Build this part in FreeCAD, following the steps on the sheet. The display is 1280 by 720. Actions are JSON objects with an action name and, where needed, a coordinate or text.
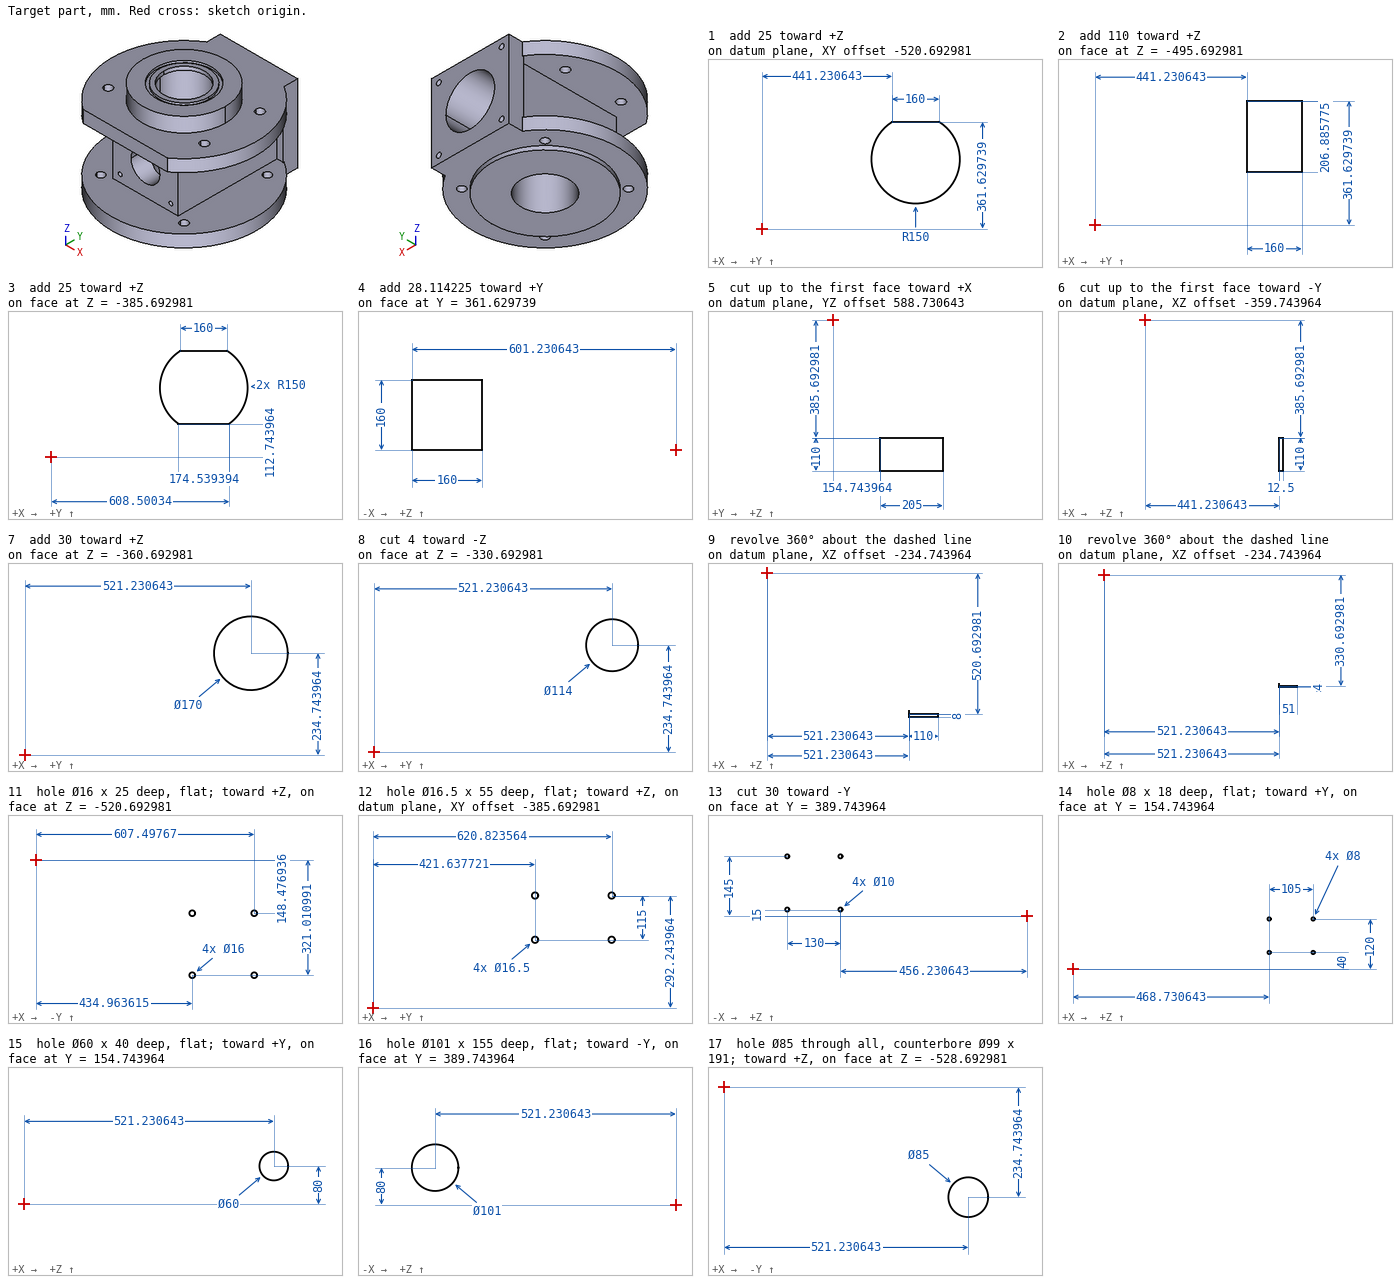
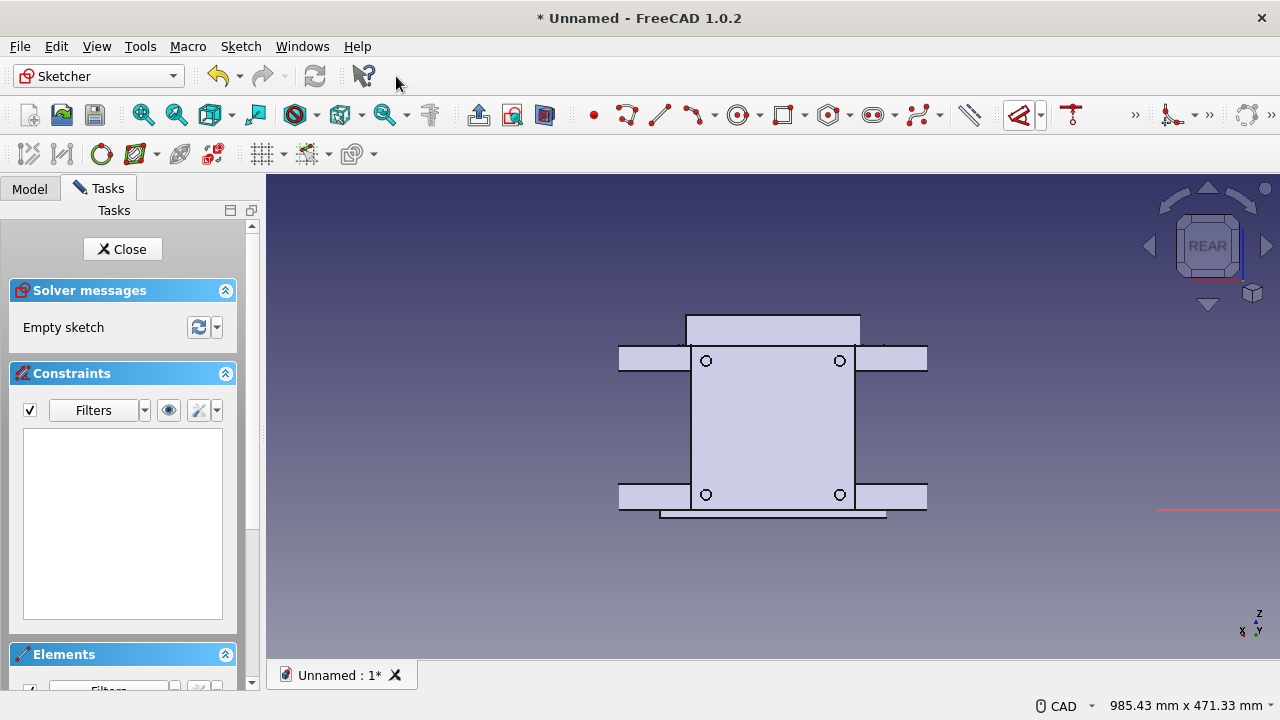
{"action": "scroll", "coordinate": [813, 434], "scroll_direction": "up", "scroll_amount": 5}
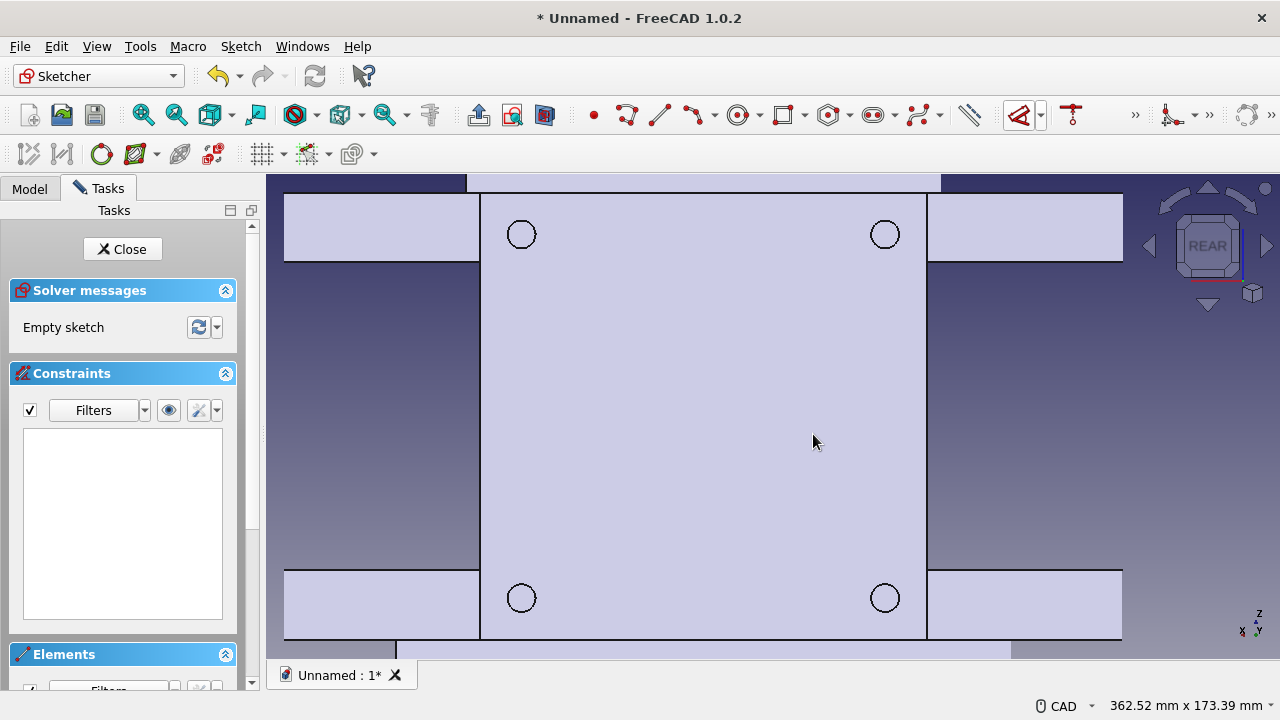
{"action": "left_click", "coordinate": [738, 116]}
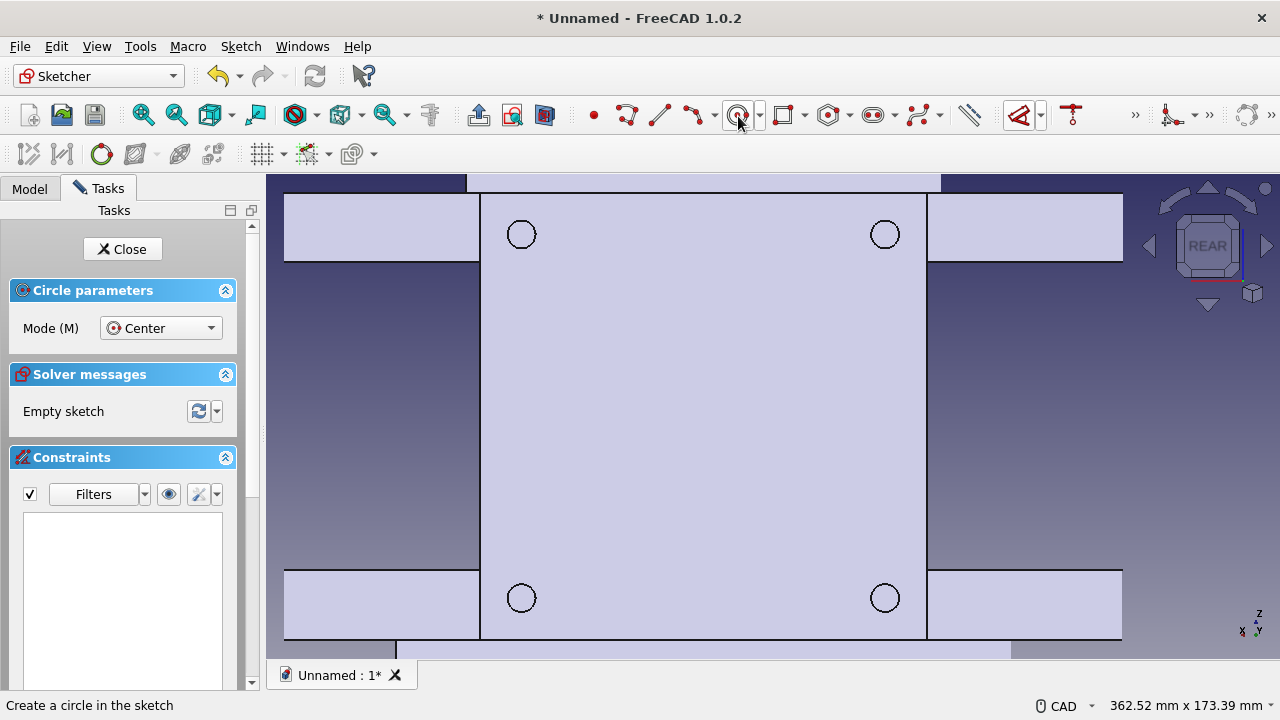
{"action": "left_click", "coordinate": [703, 416]}
{"action": "left_click", "coordinate": [803, 316]}
{"action": "key", "text": "Escape"}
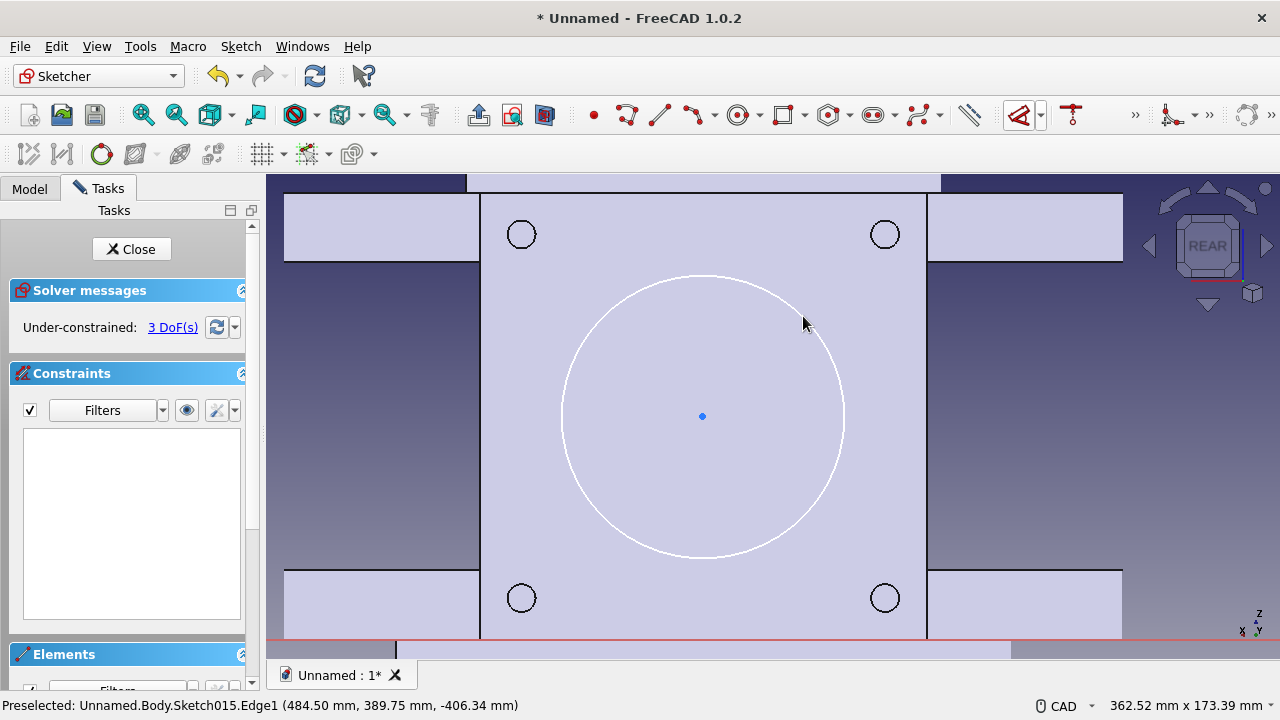
{"action": "left_click", "coordinate": [803, 317]}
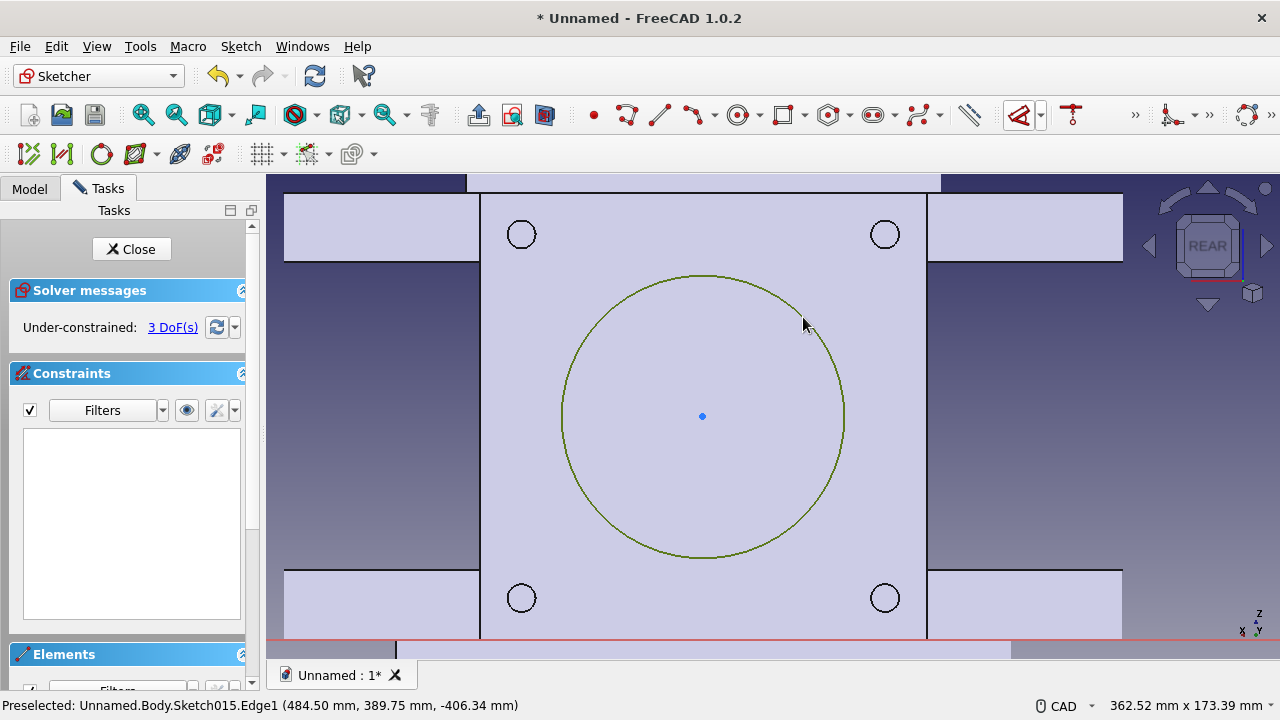
{"action": "left_click", "coordinate": [1040, 116]}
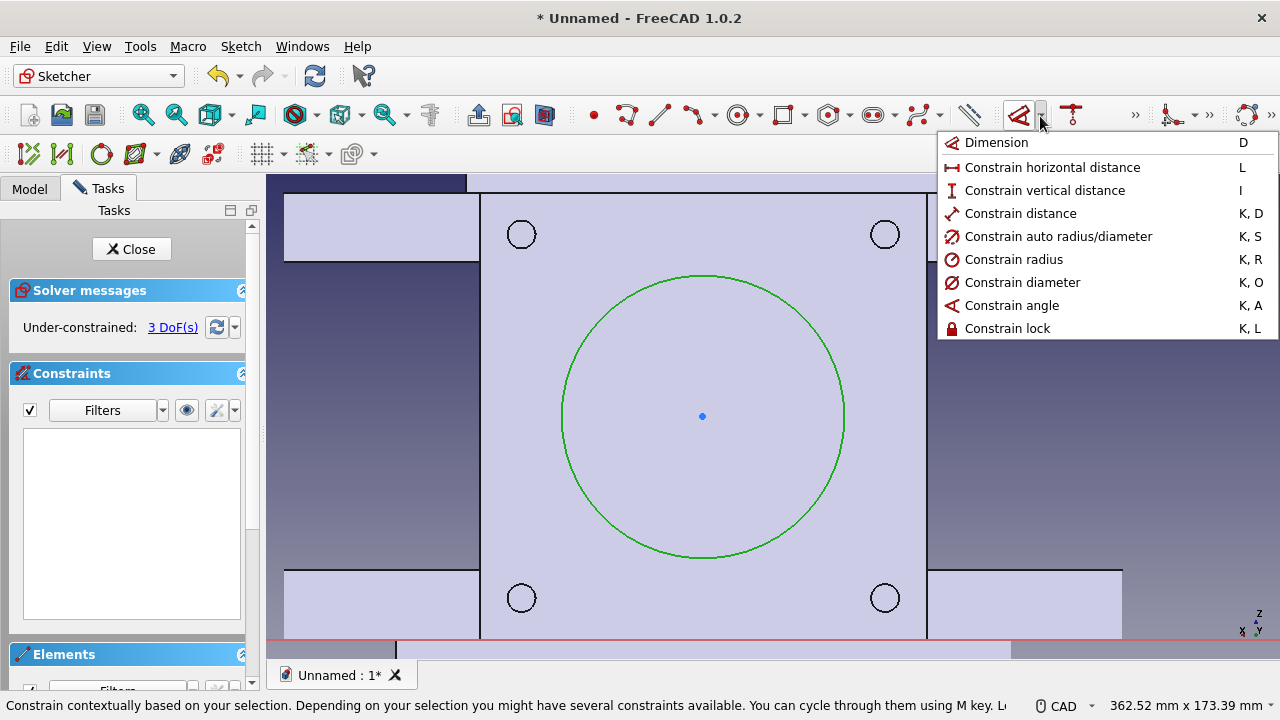
{"action": "left_click", "coordinate": [1108, 282]}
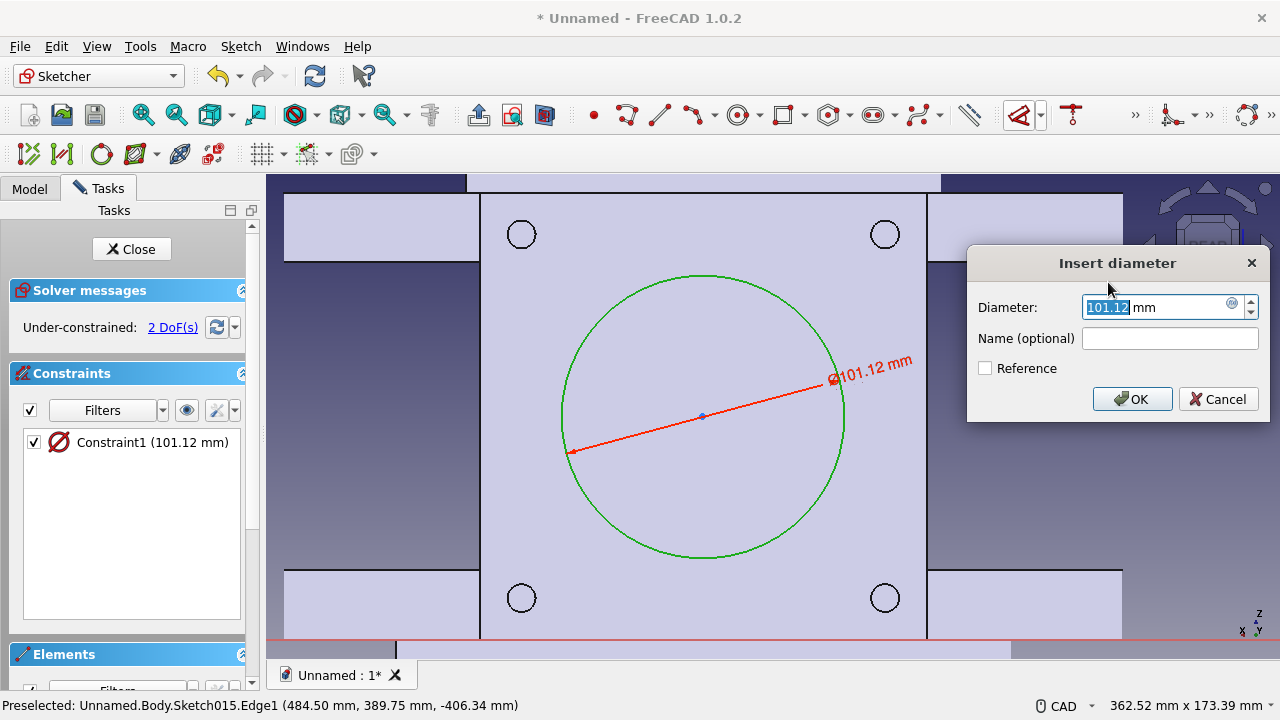
{"action": "type", "text": "101"}
{"action": "key", "text": "Return"}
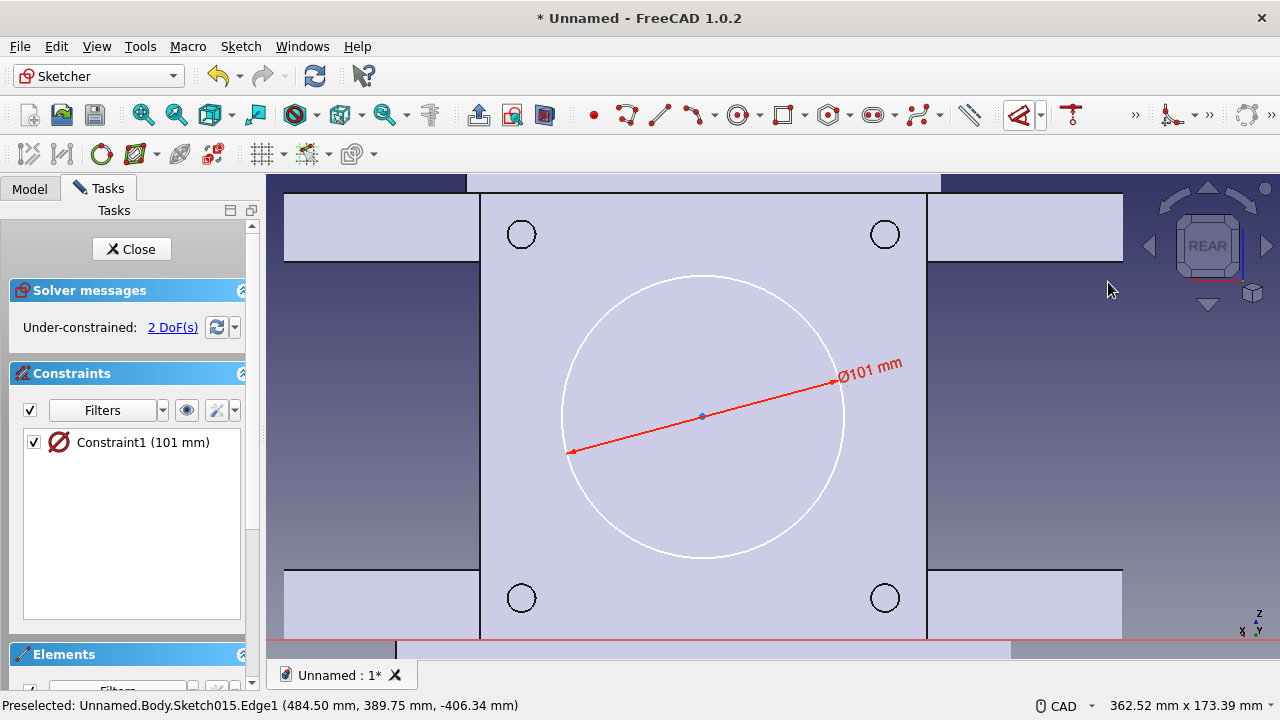
{"action": "left_click", "coordinate": [703, 417]}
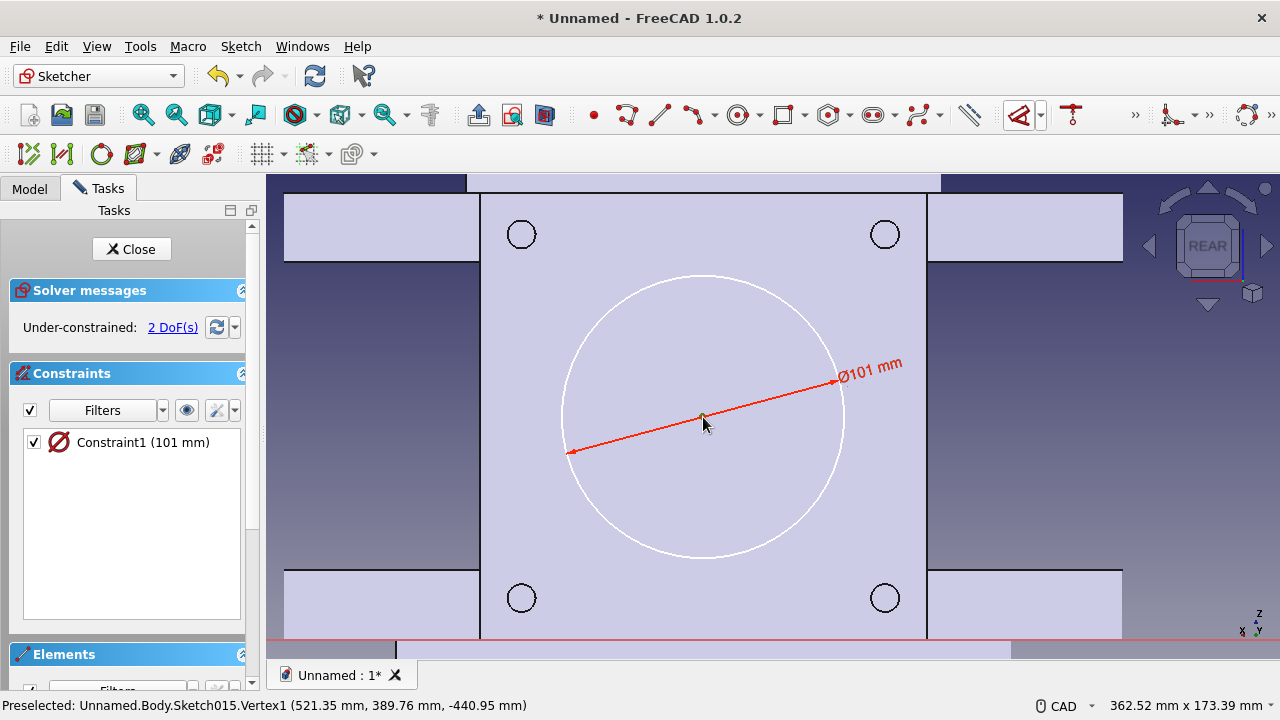
{"action": "key", "text": "i"}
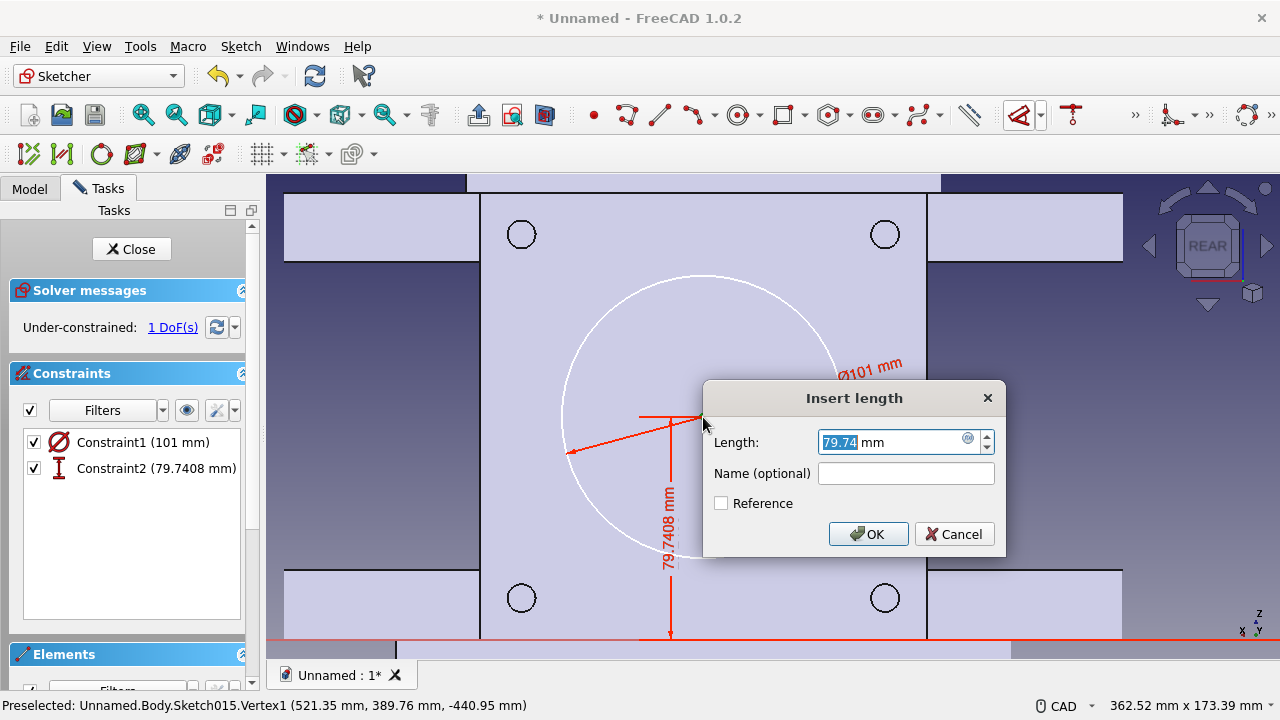
{"action": "type", "text": "80"}
{"action": "key", "text": "Return"}